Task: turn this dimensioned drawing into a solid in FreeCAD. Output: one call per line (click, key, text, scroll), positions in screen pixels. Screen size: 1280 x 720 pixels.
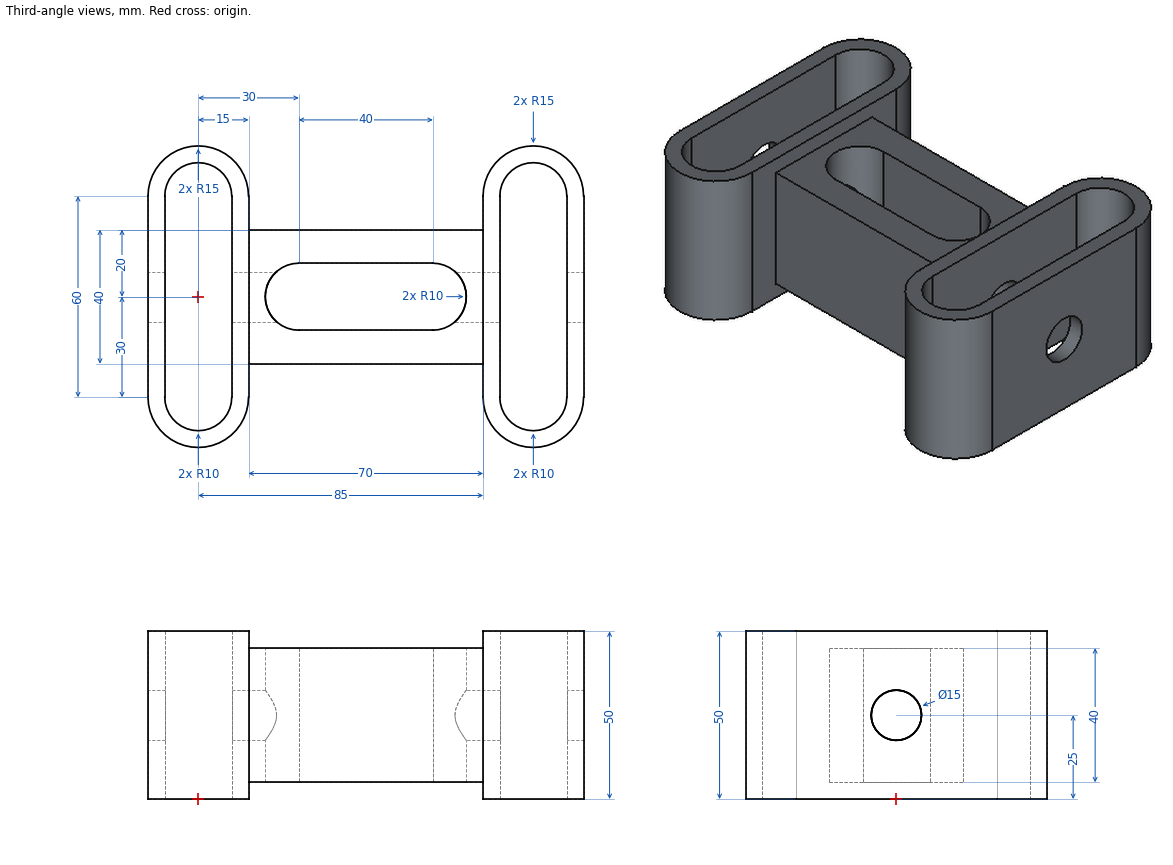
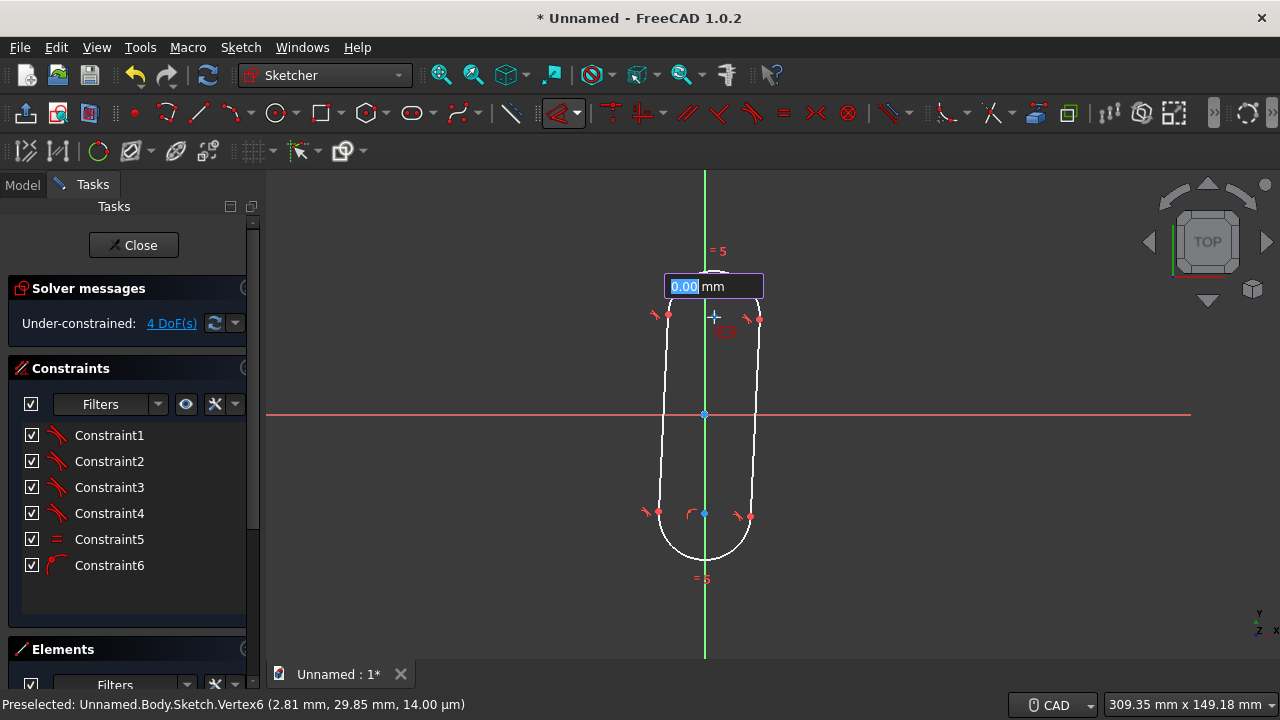
click(738, 385)
key(Escape)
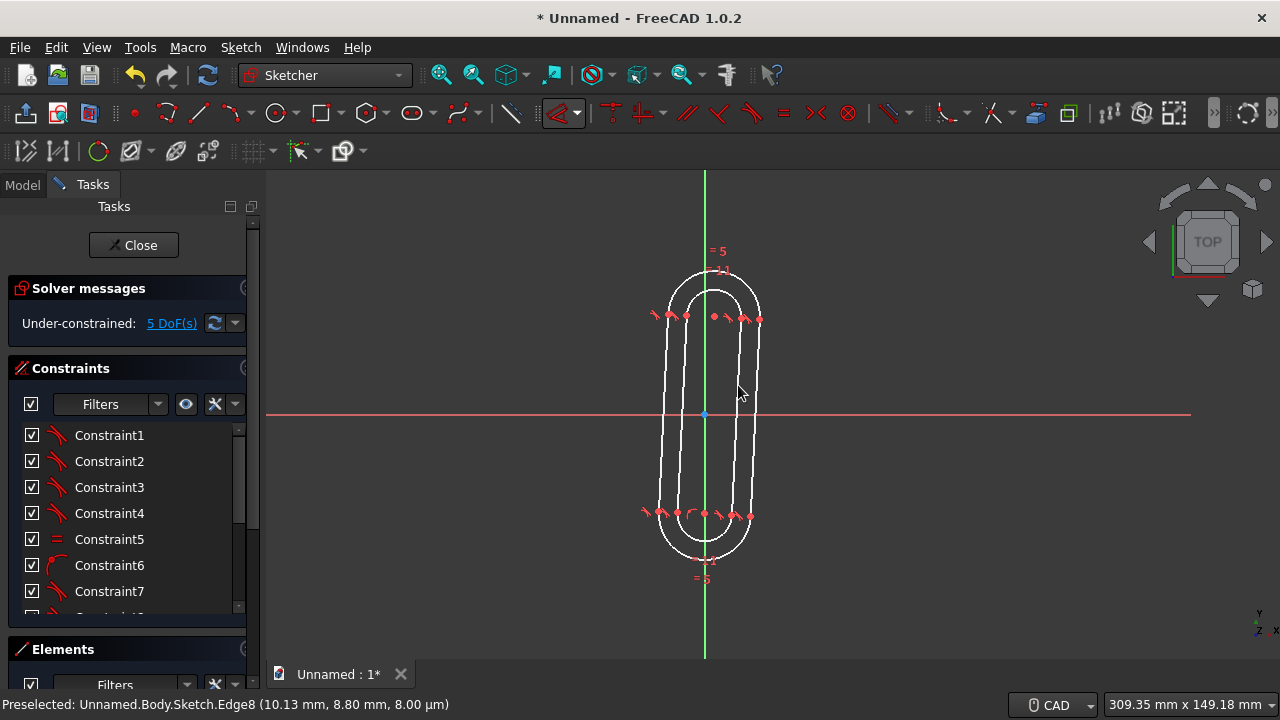
click(662, 453)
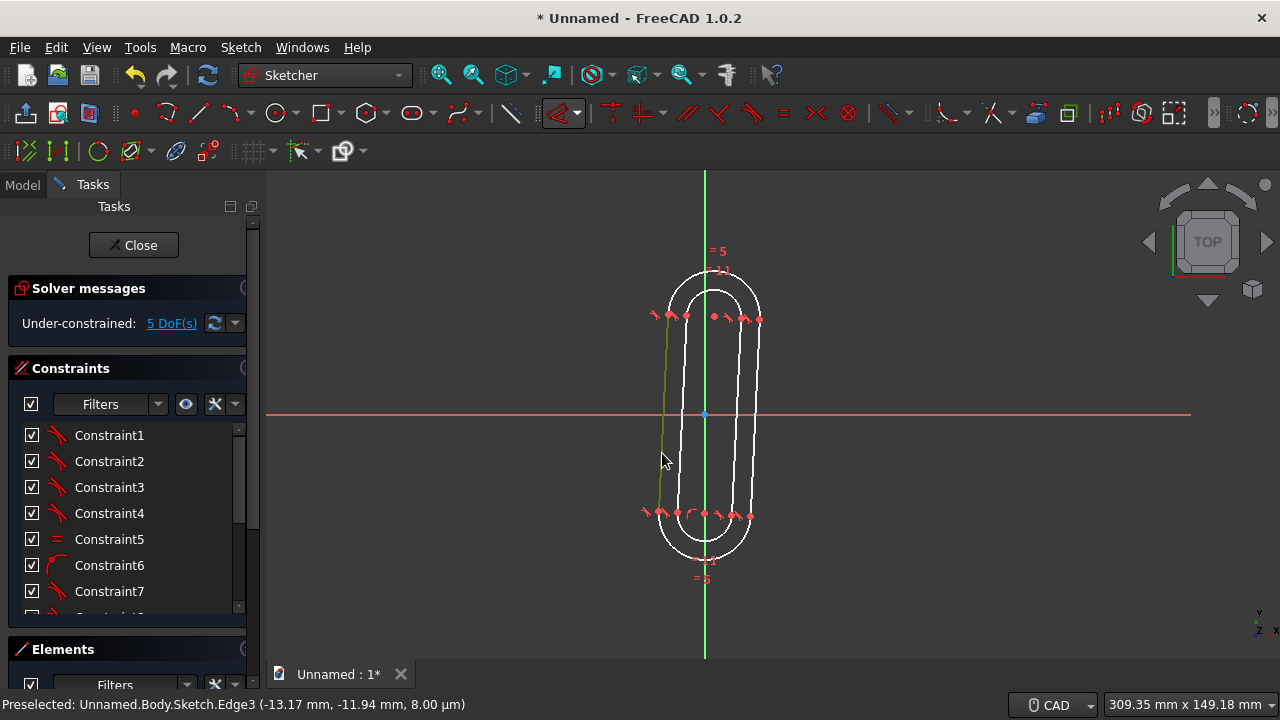
click(666, 114)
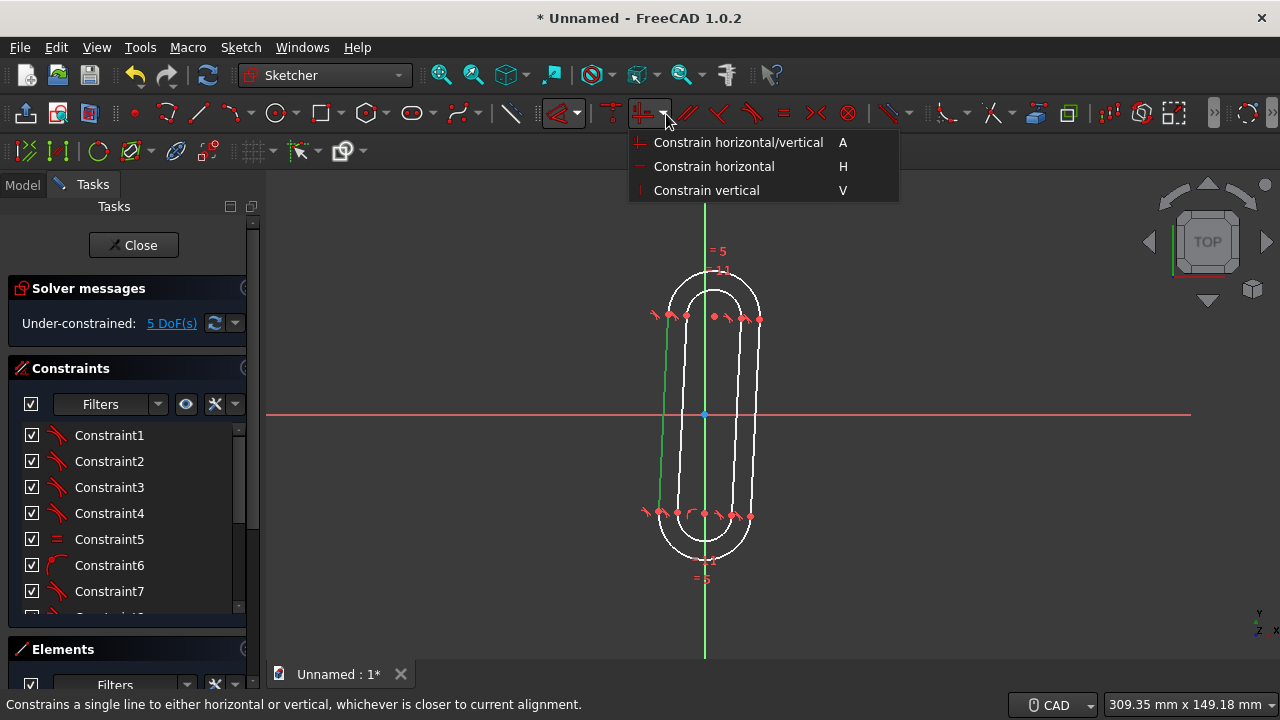
click(764, 190)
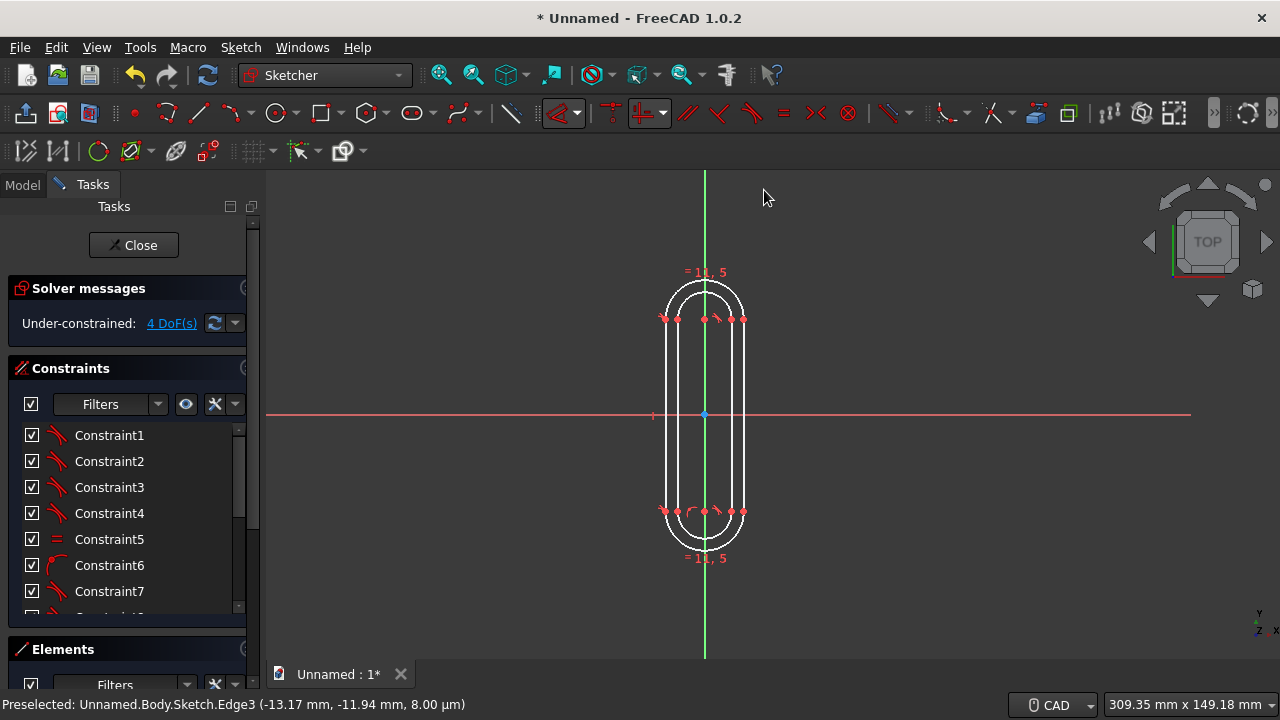
click(558, 114)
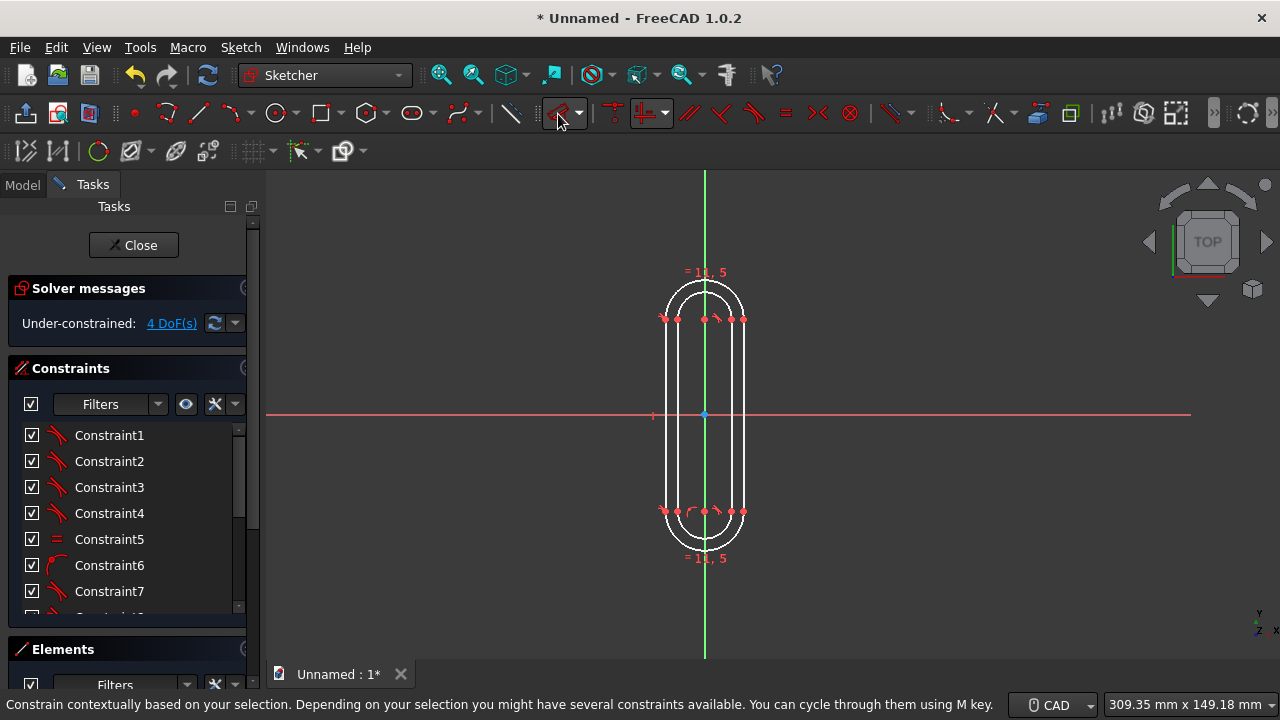
click(682, 543)
click(663, 569)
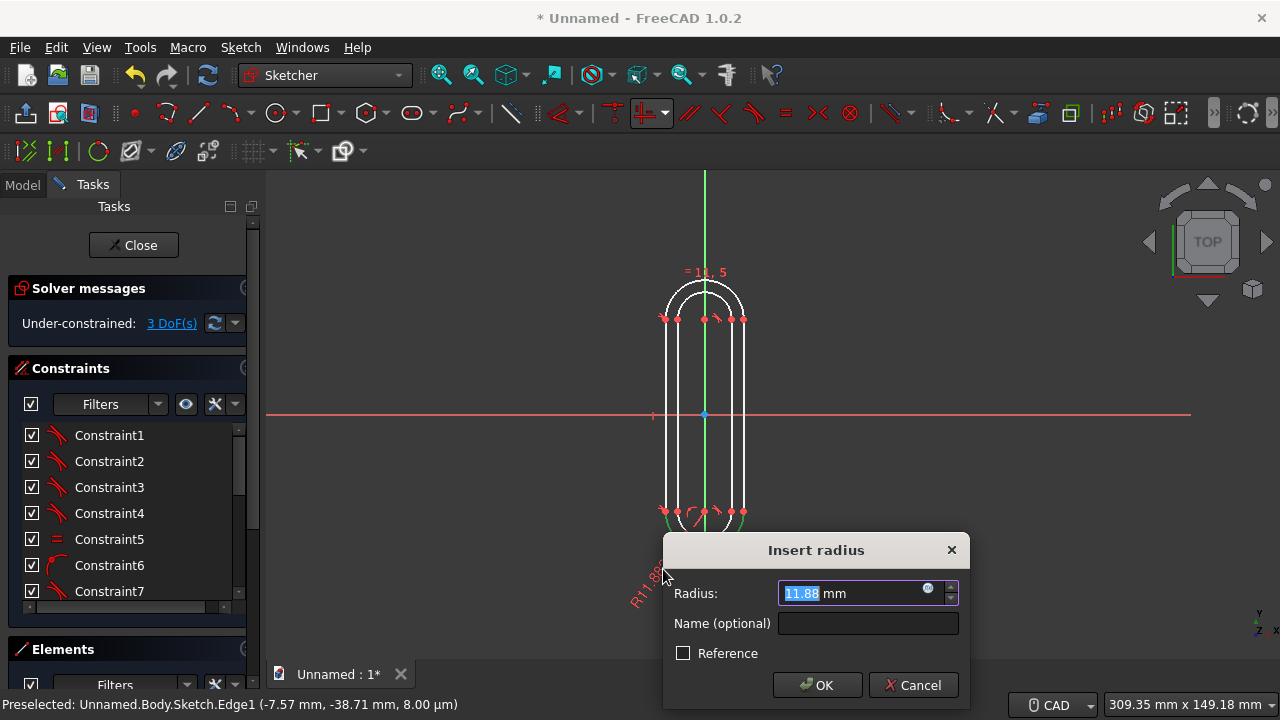
text(15)
key(Return)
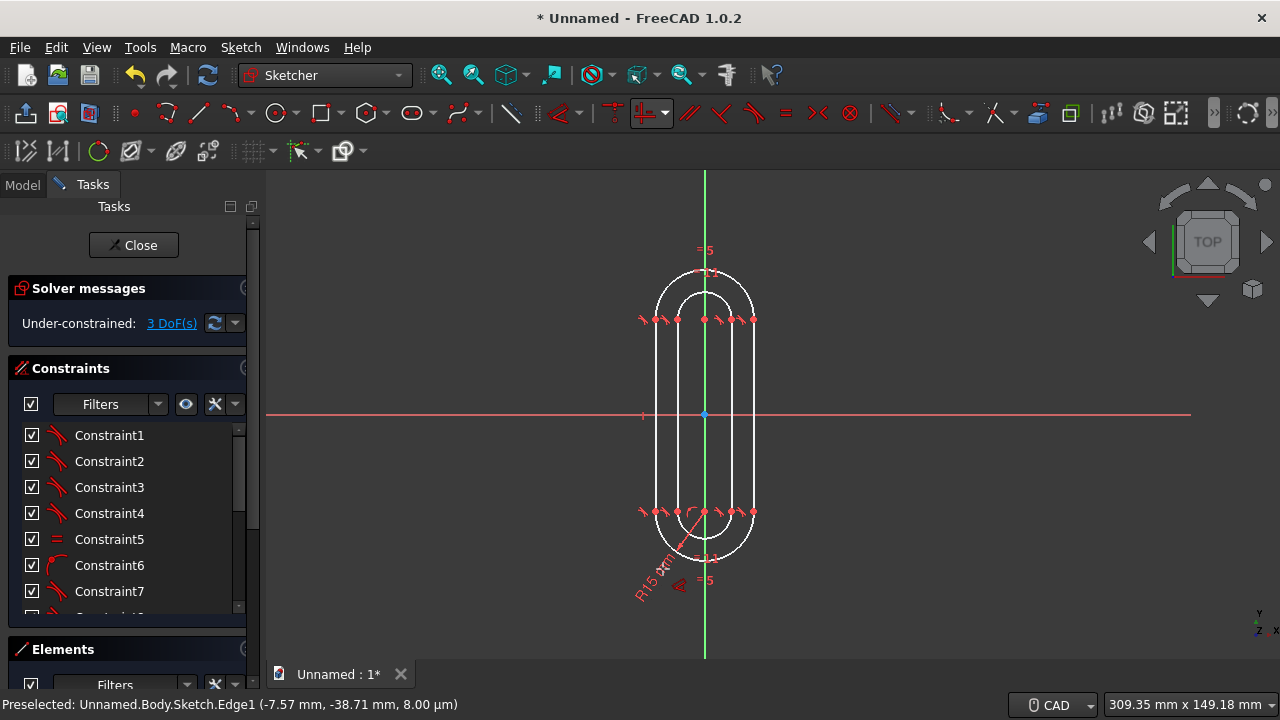
click(689, 533)
click(631, 546)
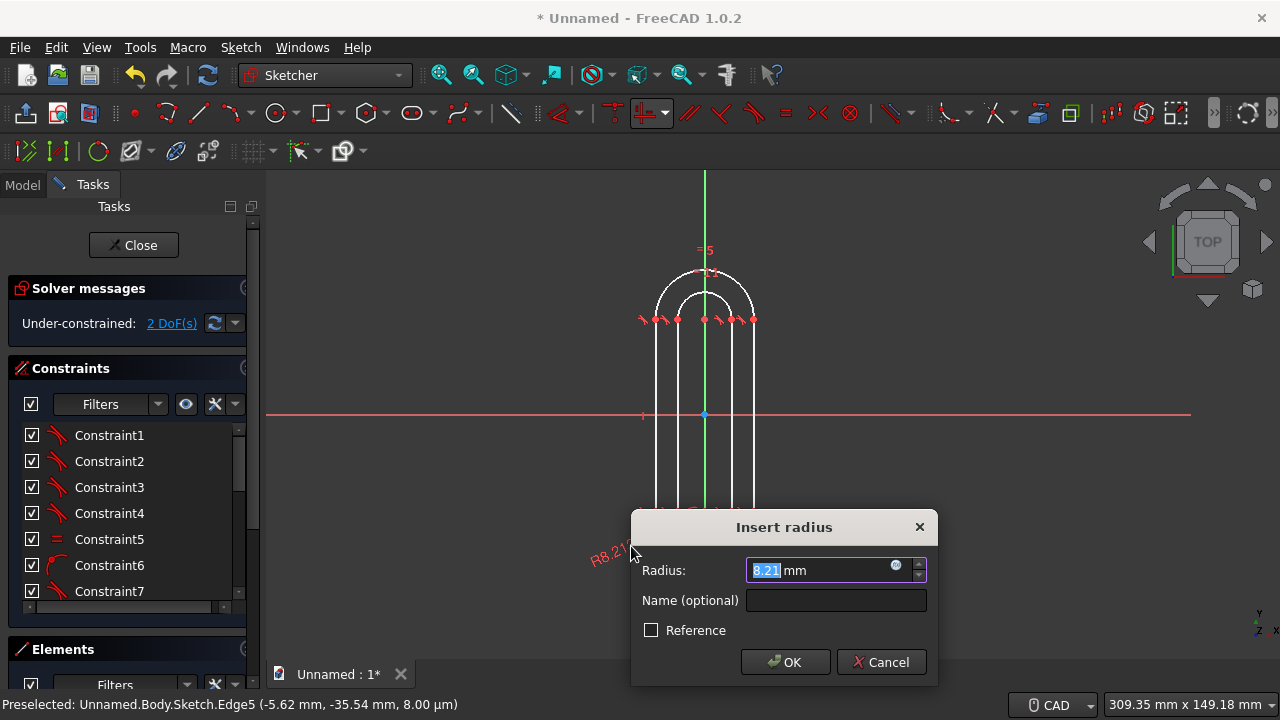
text(10)
key(Return)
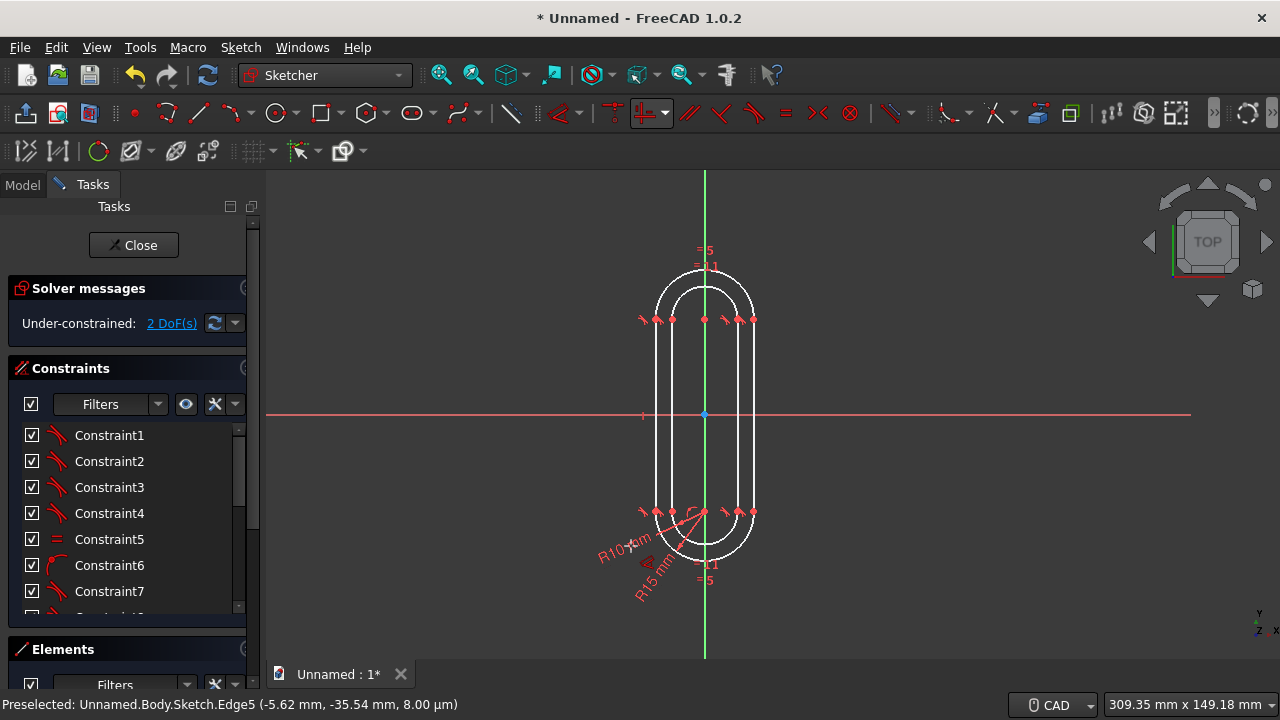
click(656, 454)
click(622, 371)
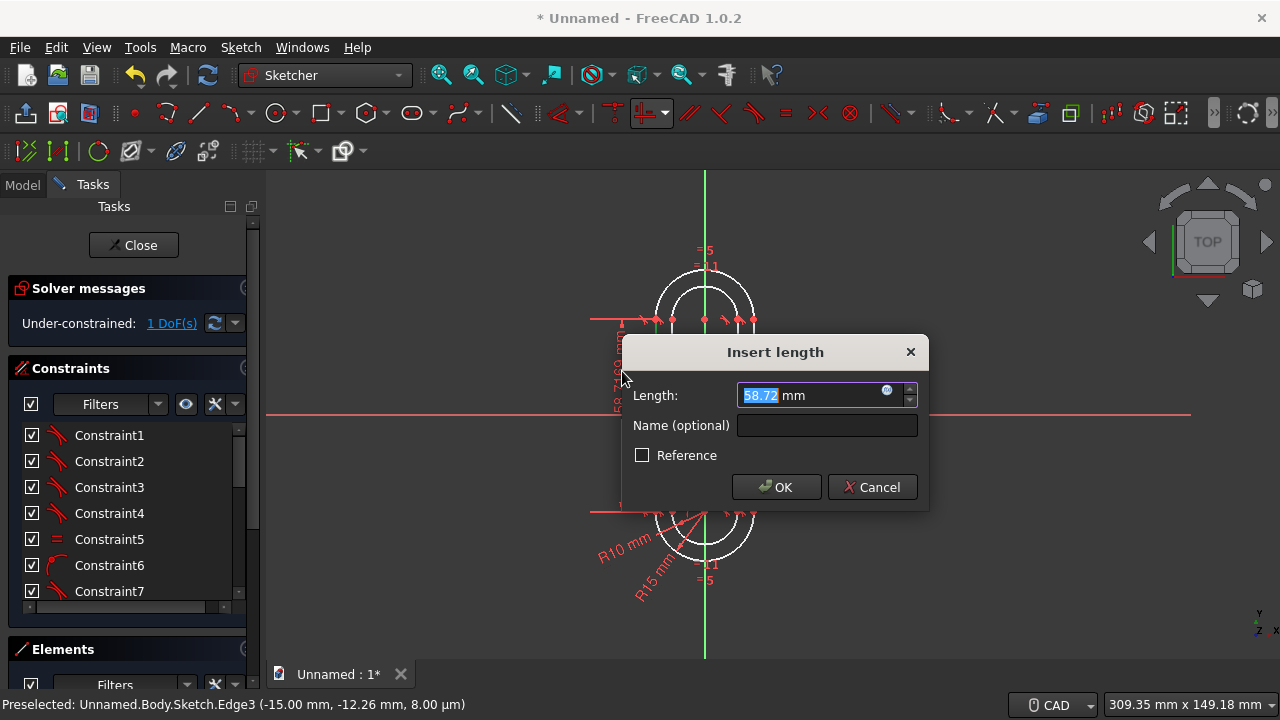
text(60)
key(Return)